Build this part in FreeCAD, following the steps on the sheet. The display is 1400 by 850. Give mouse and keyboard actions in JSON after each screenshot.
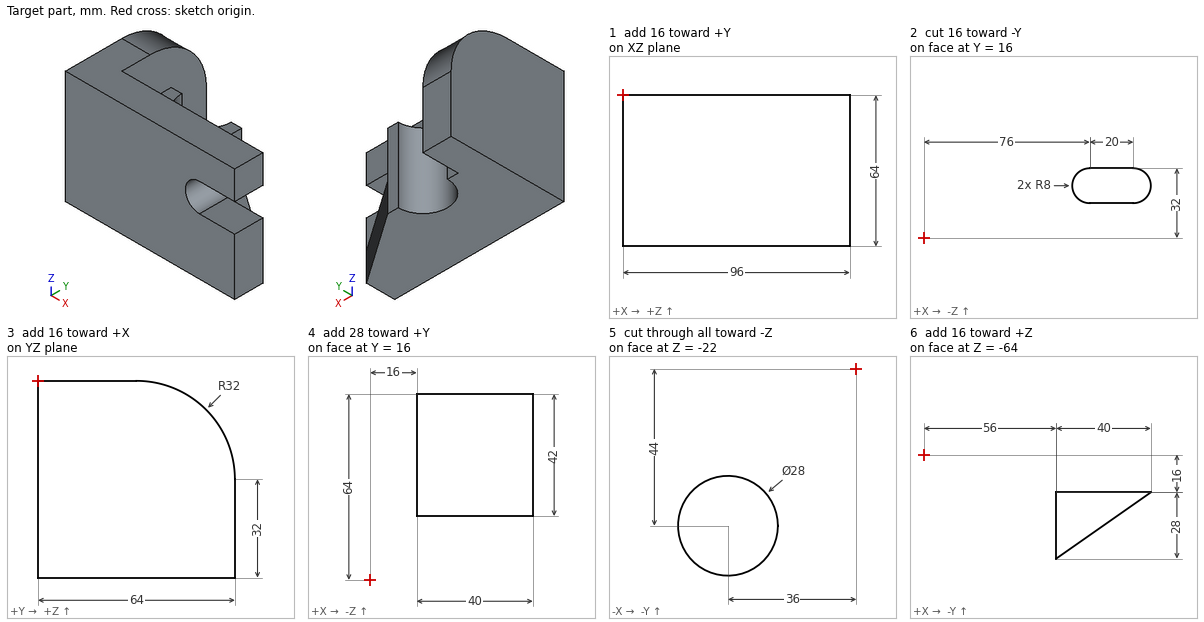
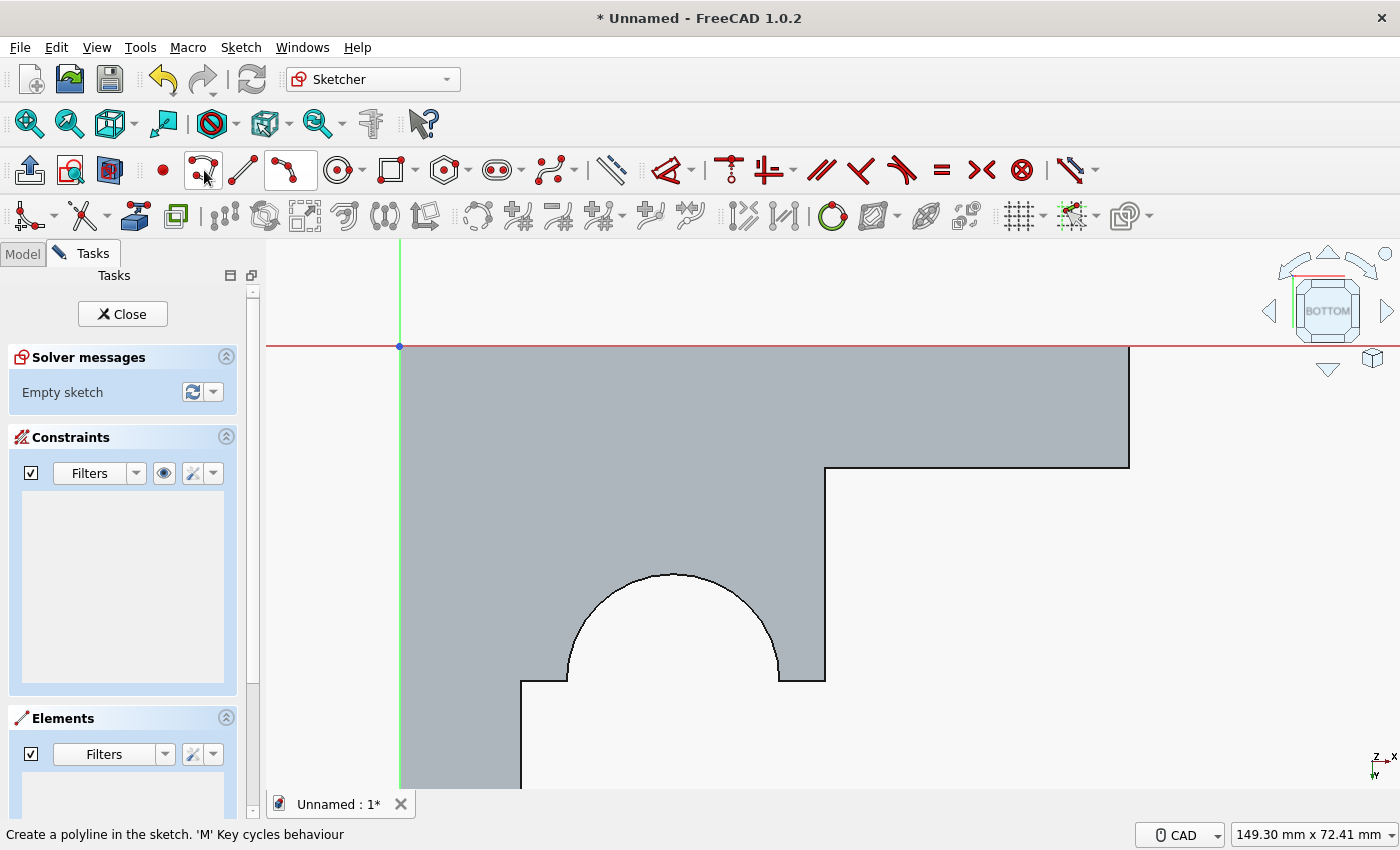
{"action": "left_click", "coordinate": [825, 468]}
{"action": "left_click", "coordinate": [825, 681]}
{"action": "left_click", "coordinate": [1129, 468]}
{"action": "left_click", "coordinate": [825, 469]}
{"action": "key", "text": "Escape"}
{"action": "key", "text": "Escape"}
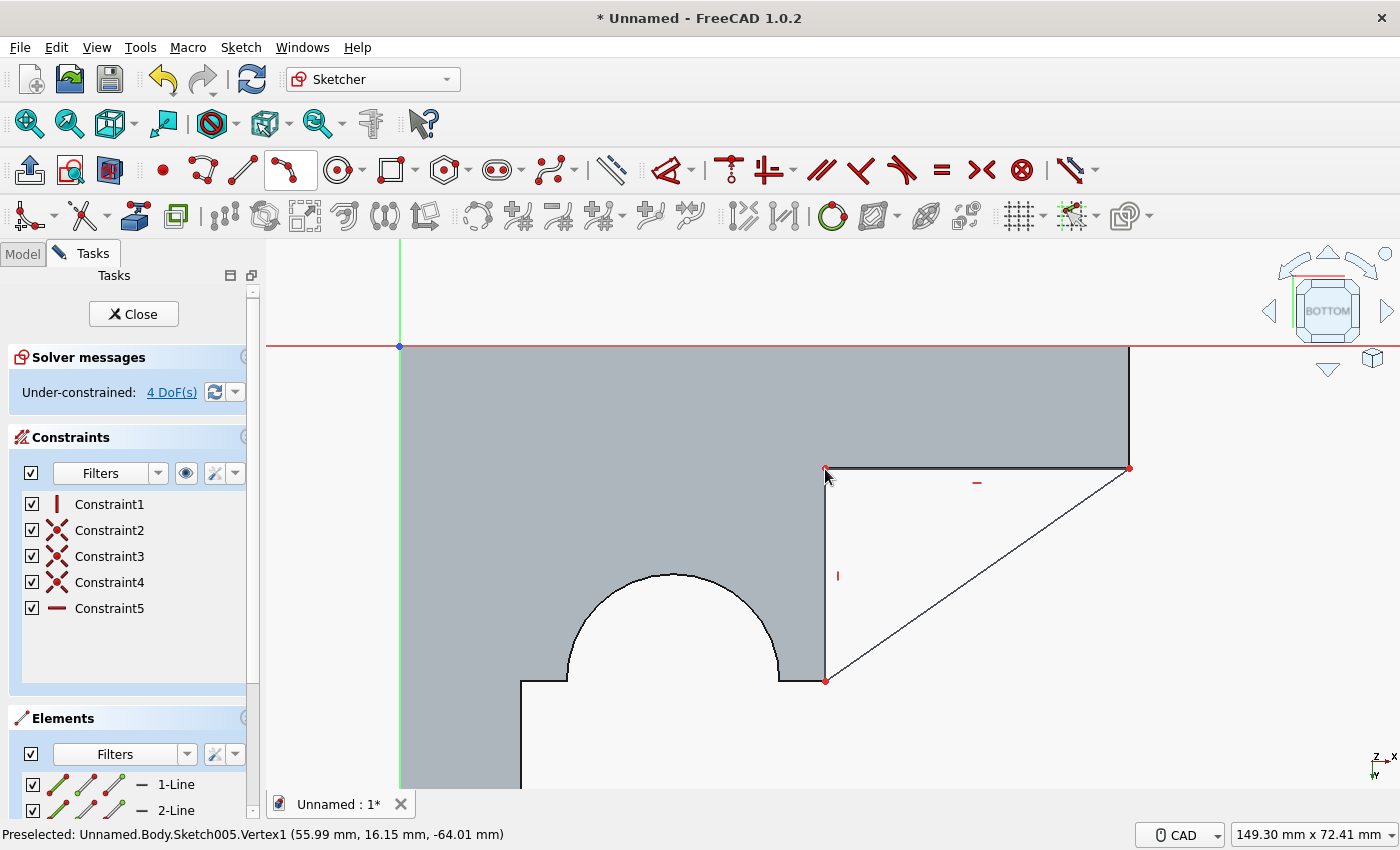
{"action": "left_click", "coordinate": [666, 170]}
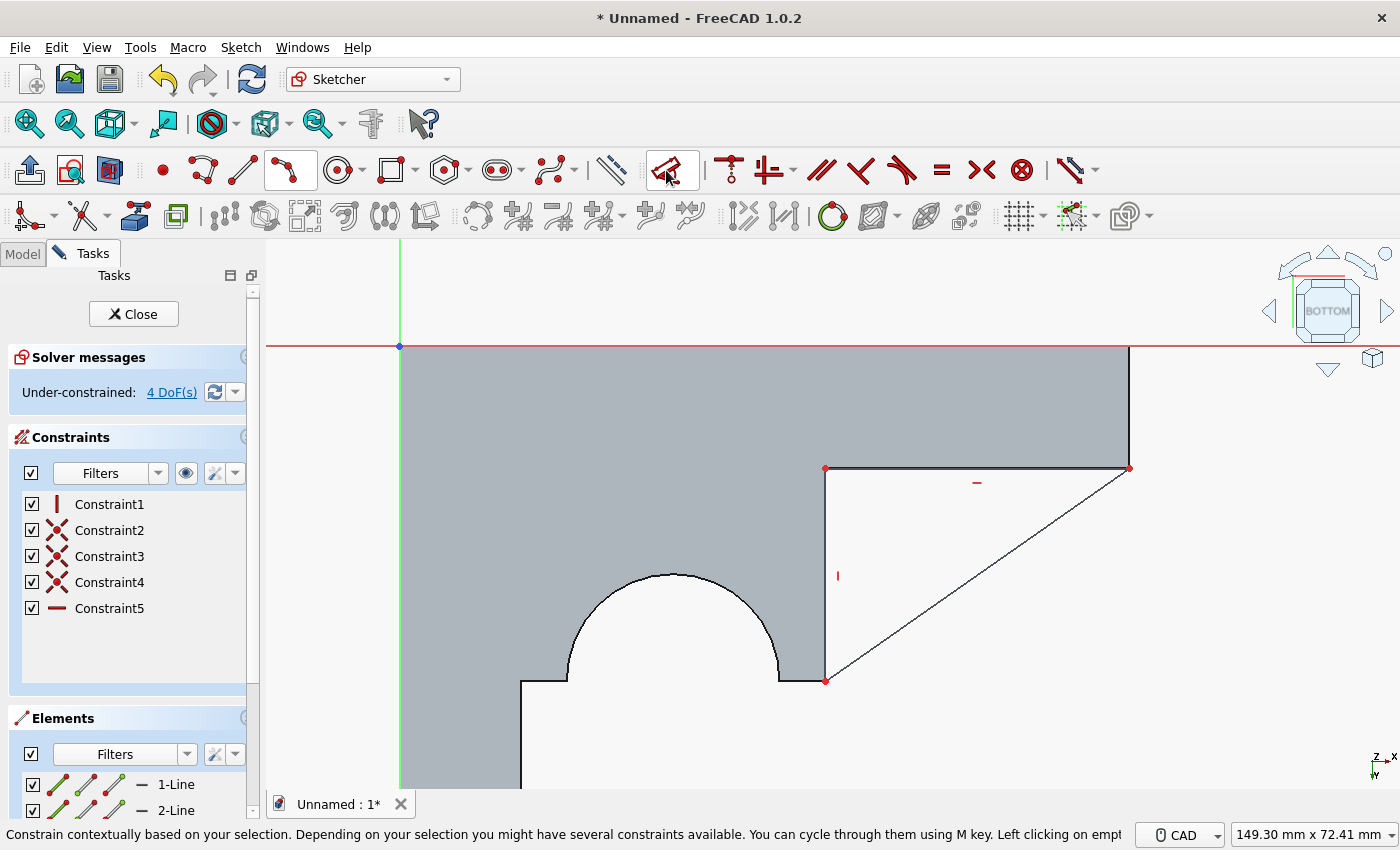
{"action": "left_click", "coordinate": [825, 533]}
{"action": "left_click", "coordinate": [859, 576]}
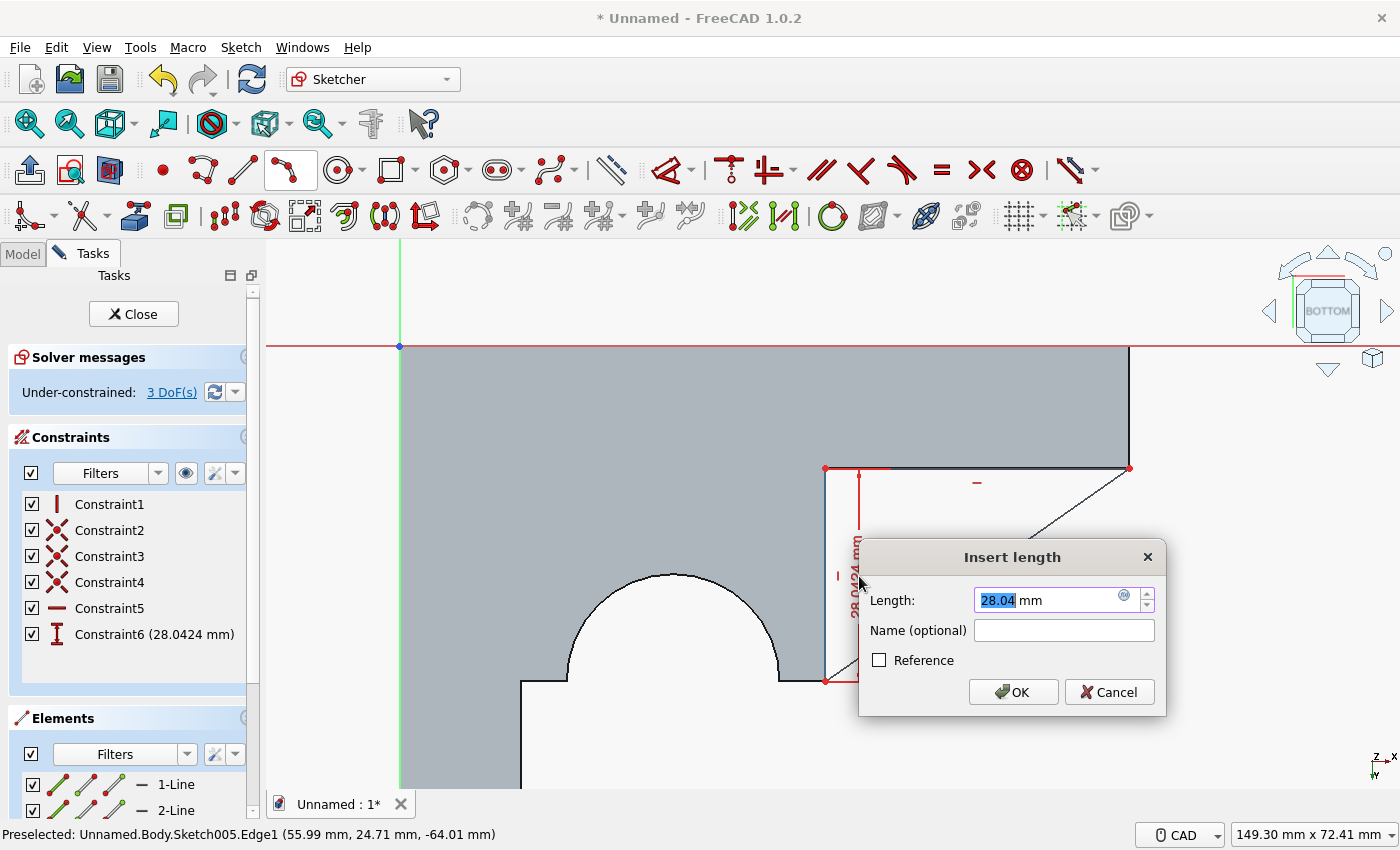
{"action": "type", "text": "28"}
{"action": "key", "text": "Return"}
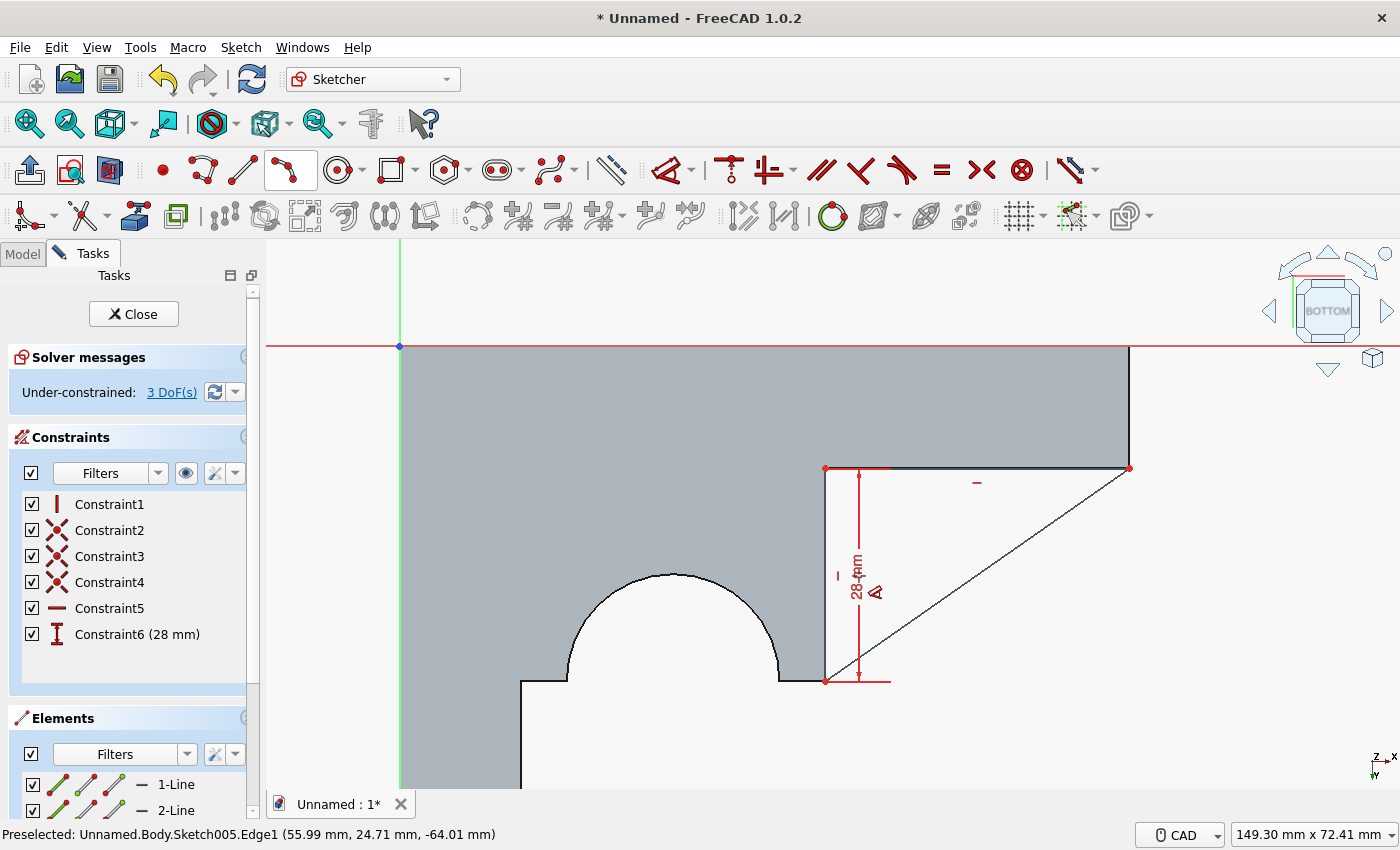
{"action": "left_click", "coordinate": [1038, 469]}
{"action": "left_click", "coordinate": [977, 435]}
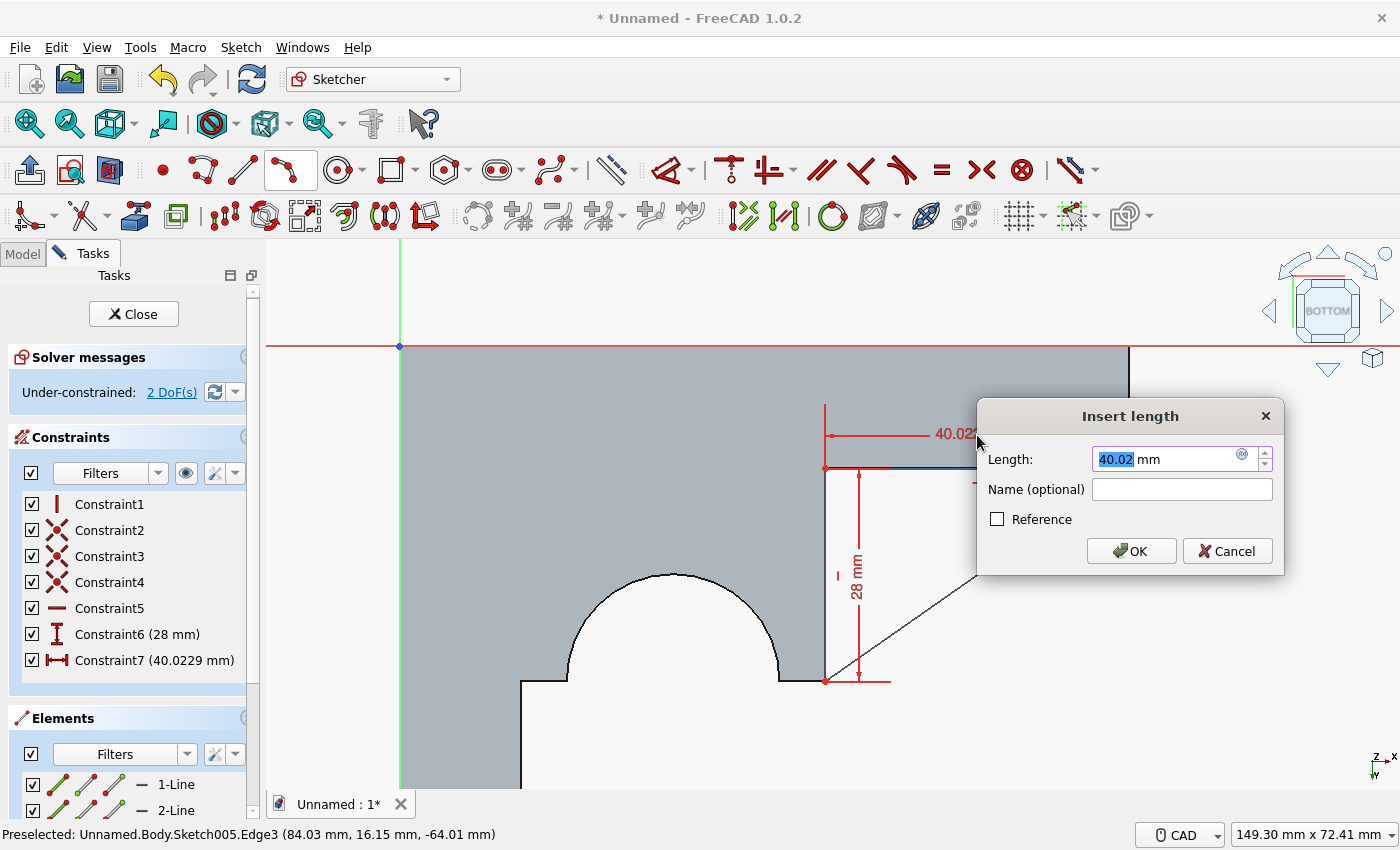
{"action": "type", "text": "40"}
{"action": "key", "text": "Return"}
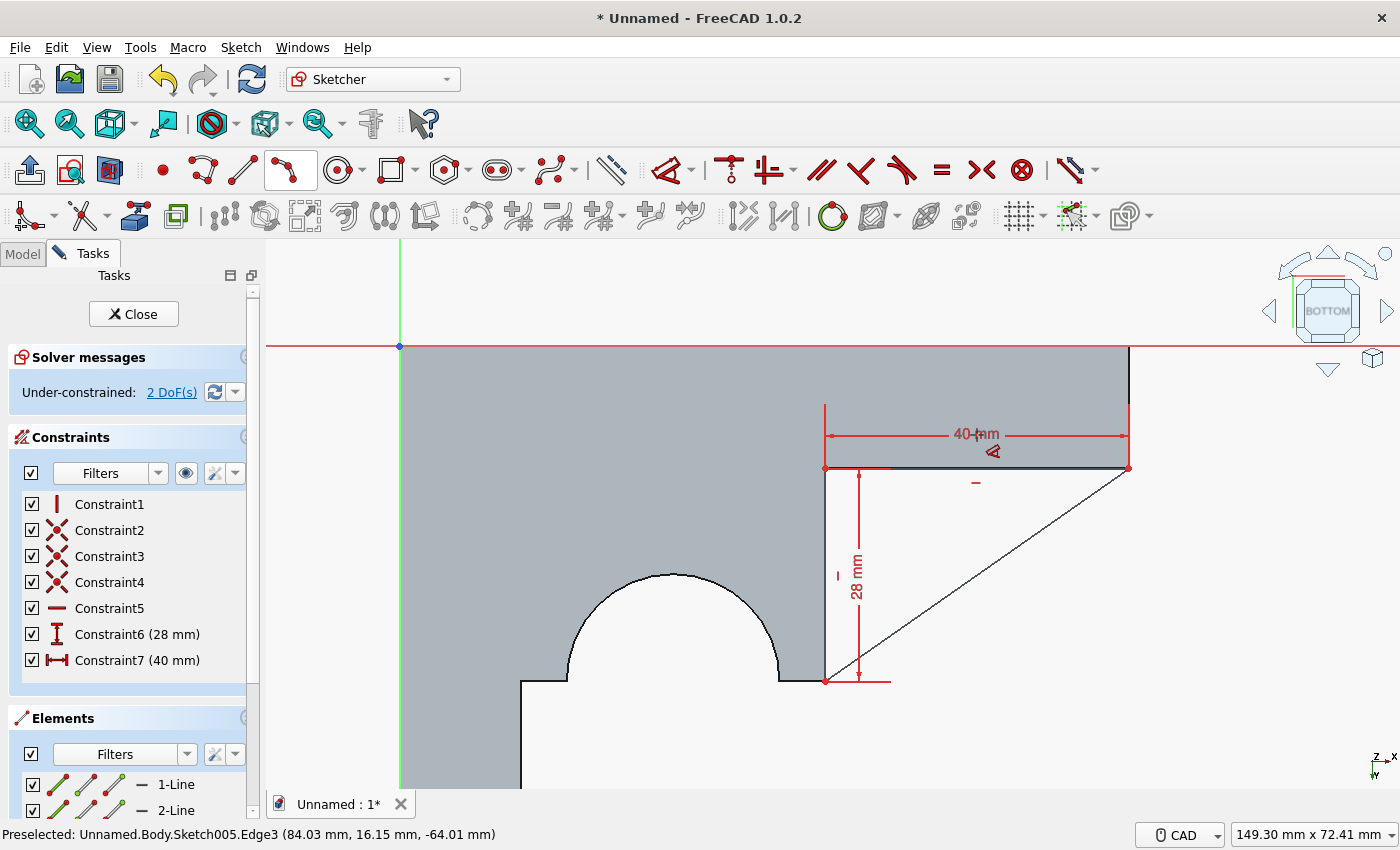
{"action": "left_click", "coordinate": [825, 469]}
{"action": "left_click", "coordinate": [612, 312]}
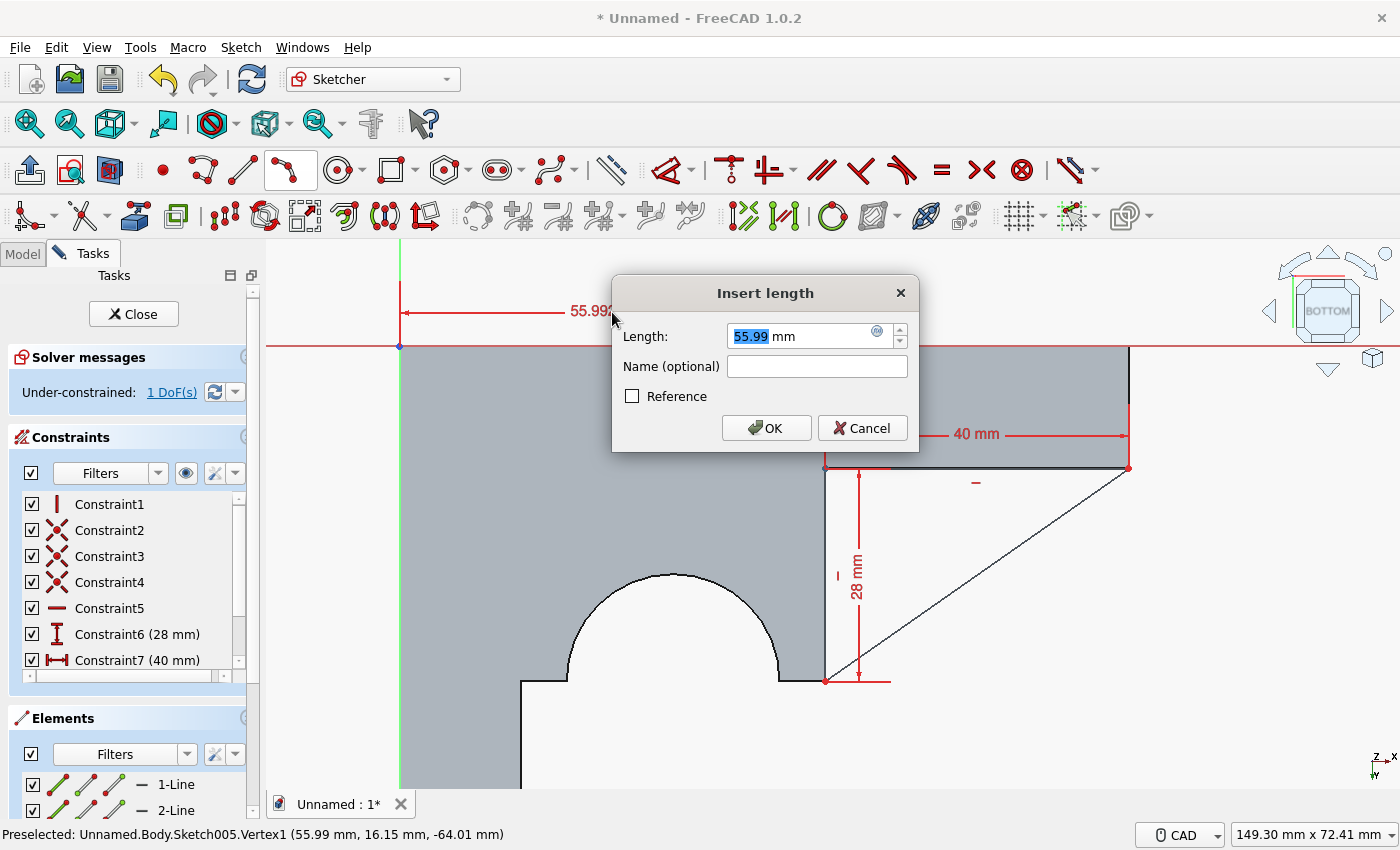
{"action": "type", "text": "56"}
{"action": "key", "text": "Return"}